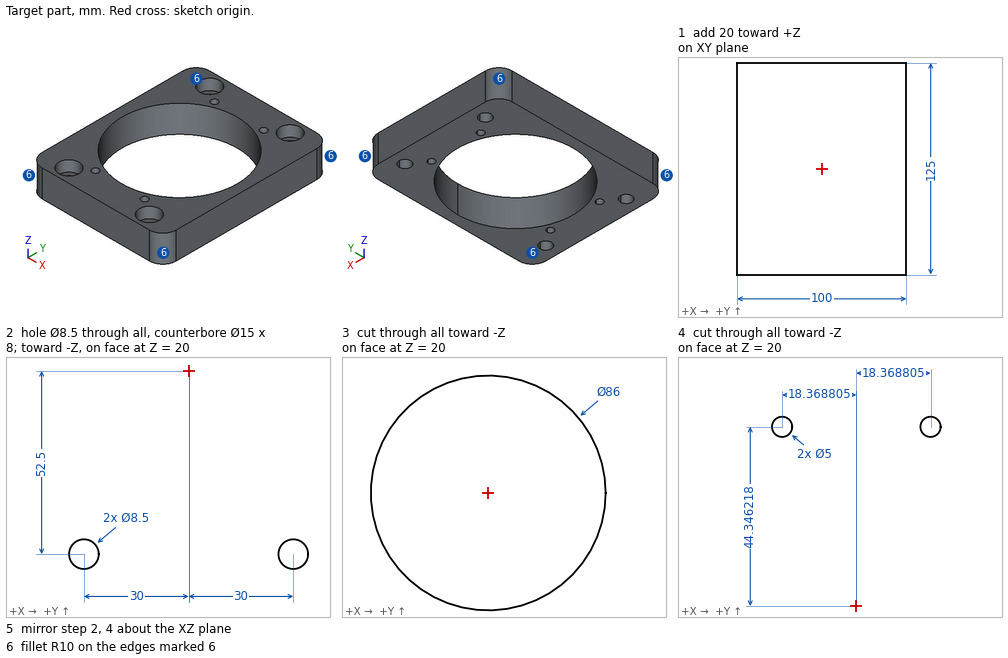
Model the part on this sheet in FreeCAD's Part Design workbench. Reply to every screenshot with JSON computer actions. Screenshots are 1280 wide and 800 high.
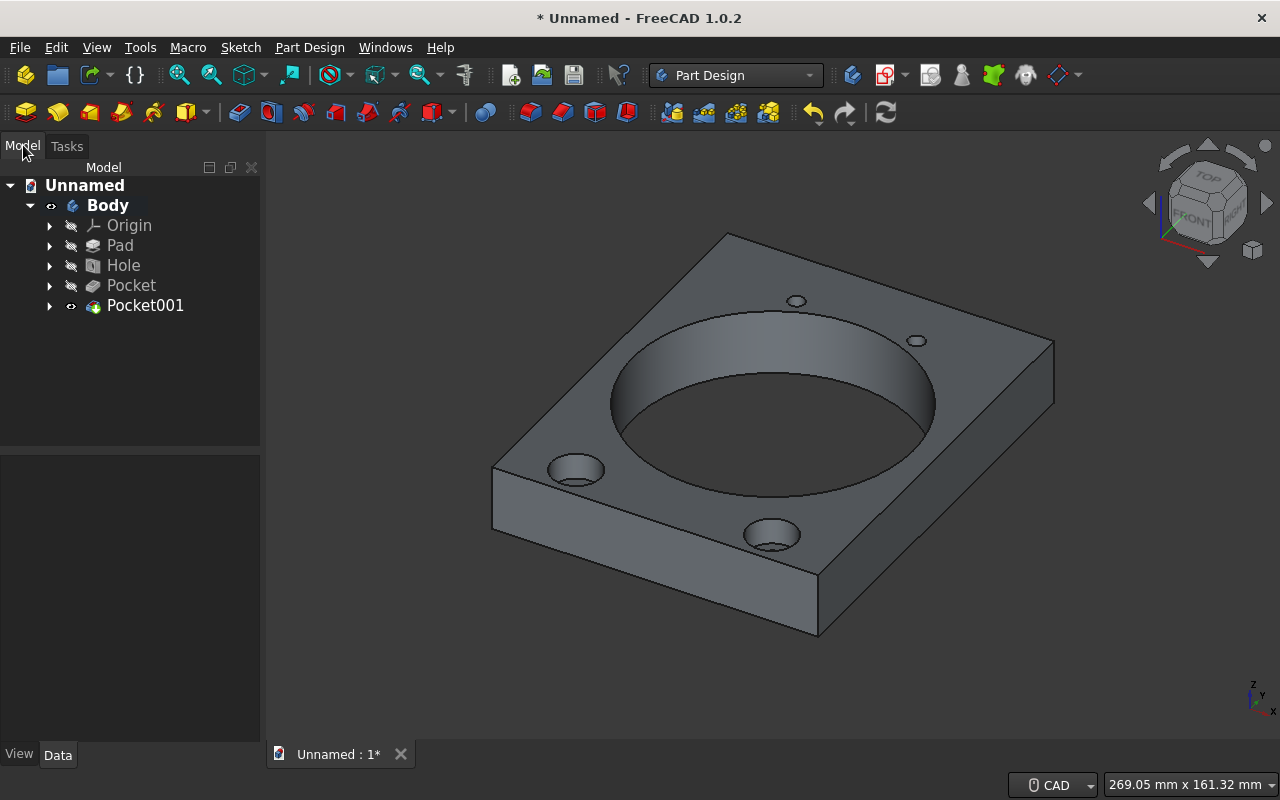
{"action": "left_click", "coordinate": [116, 266]}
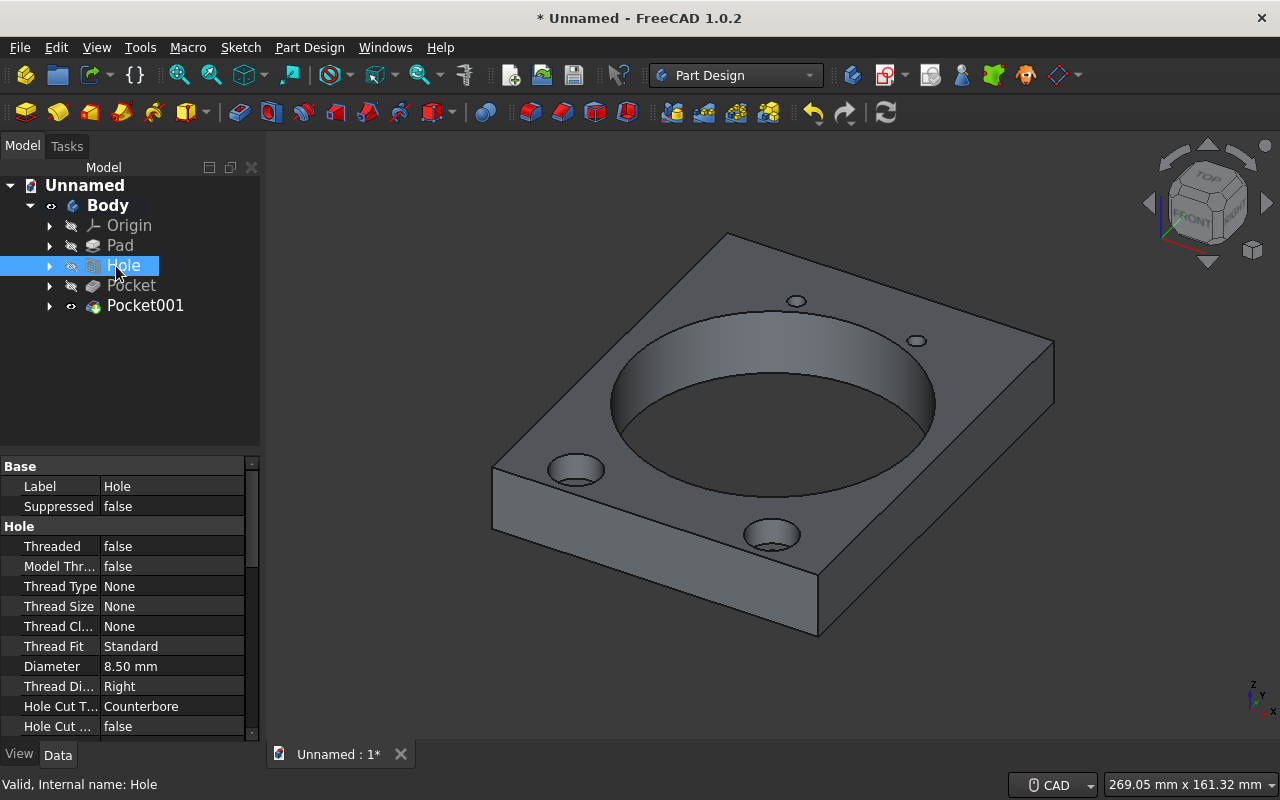
{"action": "left_click", "coordinate": [116, 306], "text": "ctrl"}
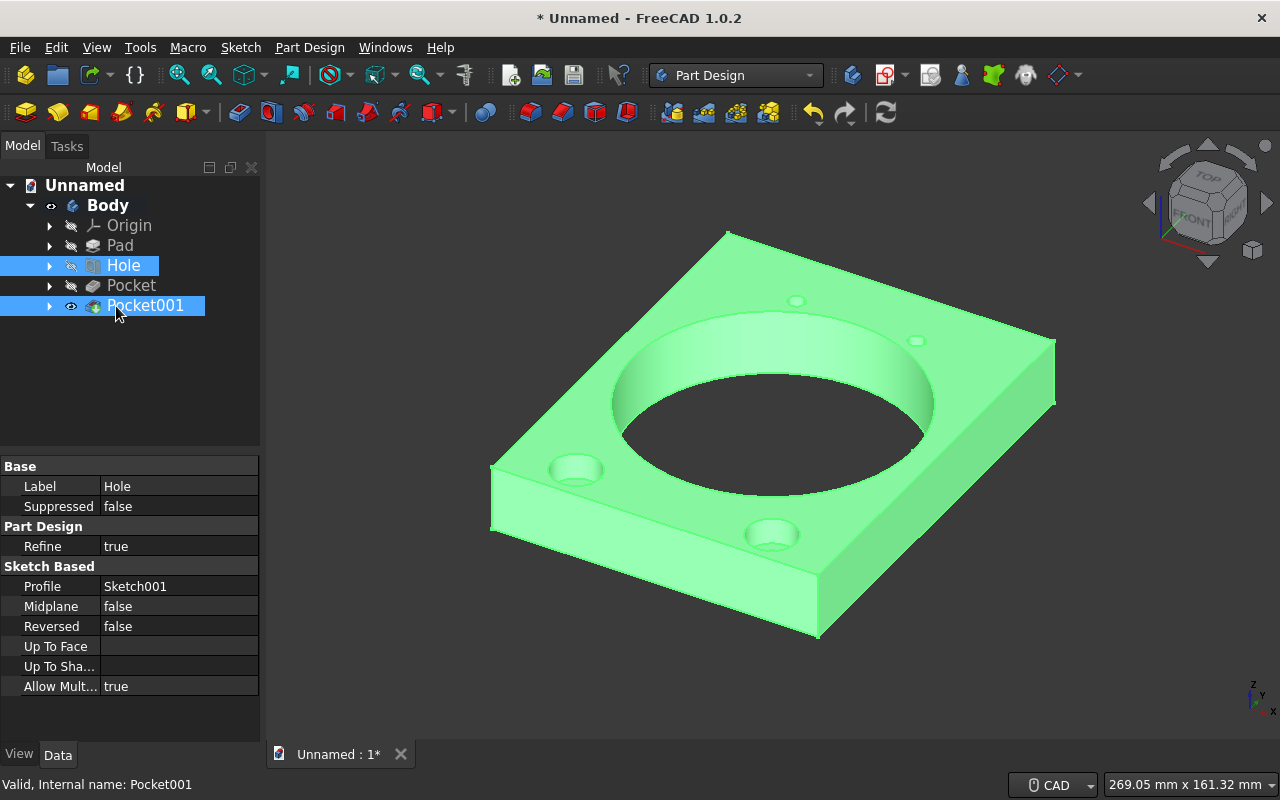
{"action": "left_click", "coordinate": [672, 112]}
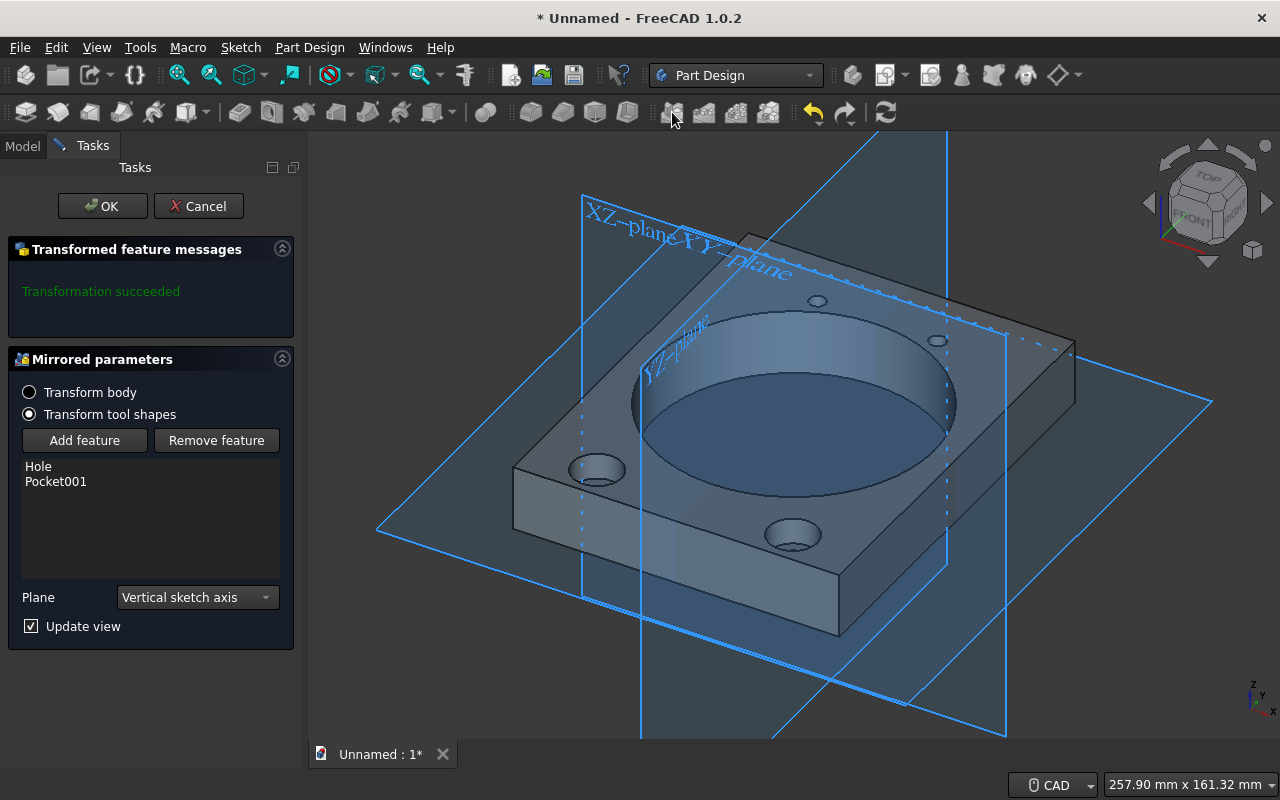
{"action": "left_click", "coordinate": [198, 598]}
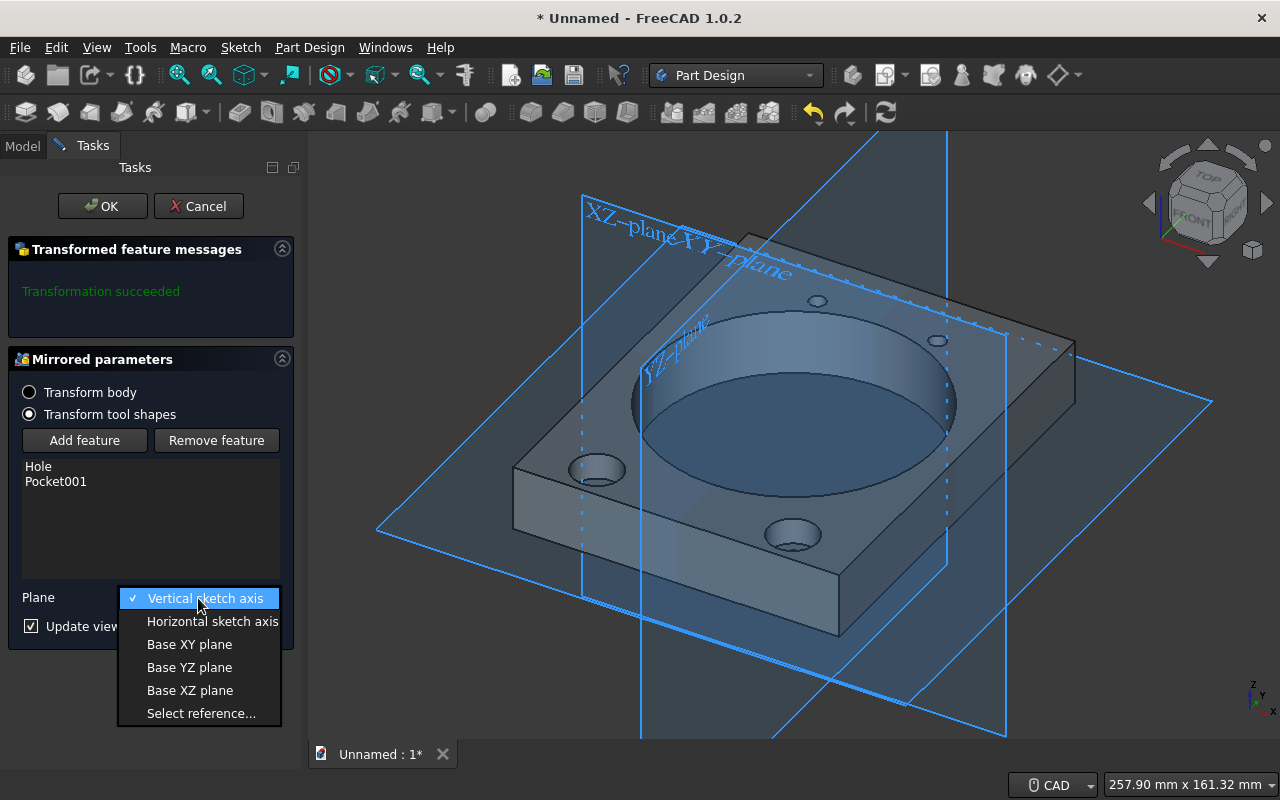
{"action": "left_click", "coordinate": [198, 690]}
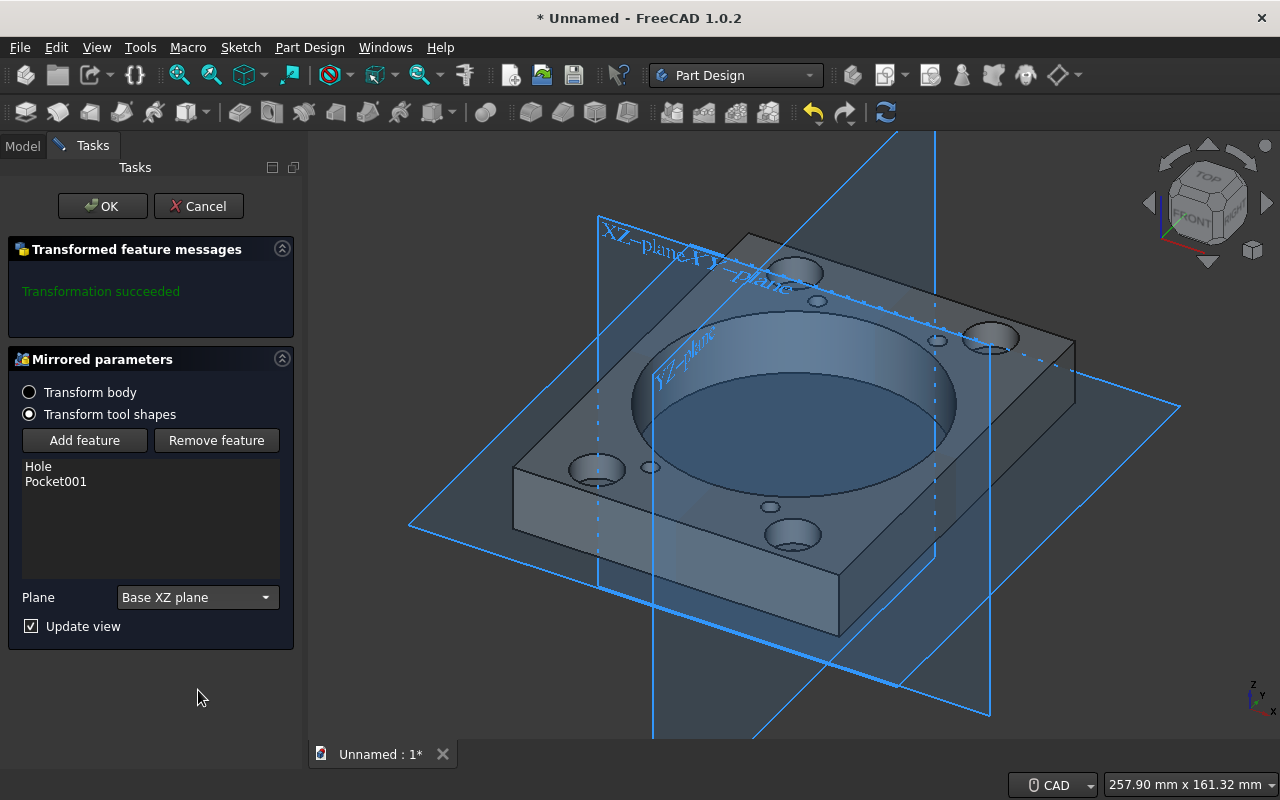
{"action": "left_click", "coordinate": [103, 206]}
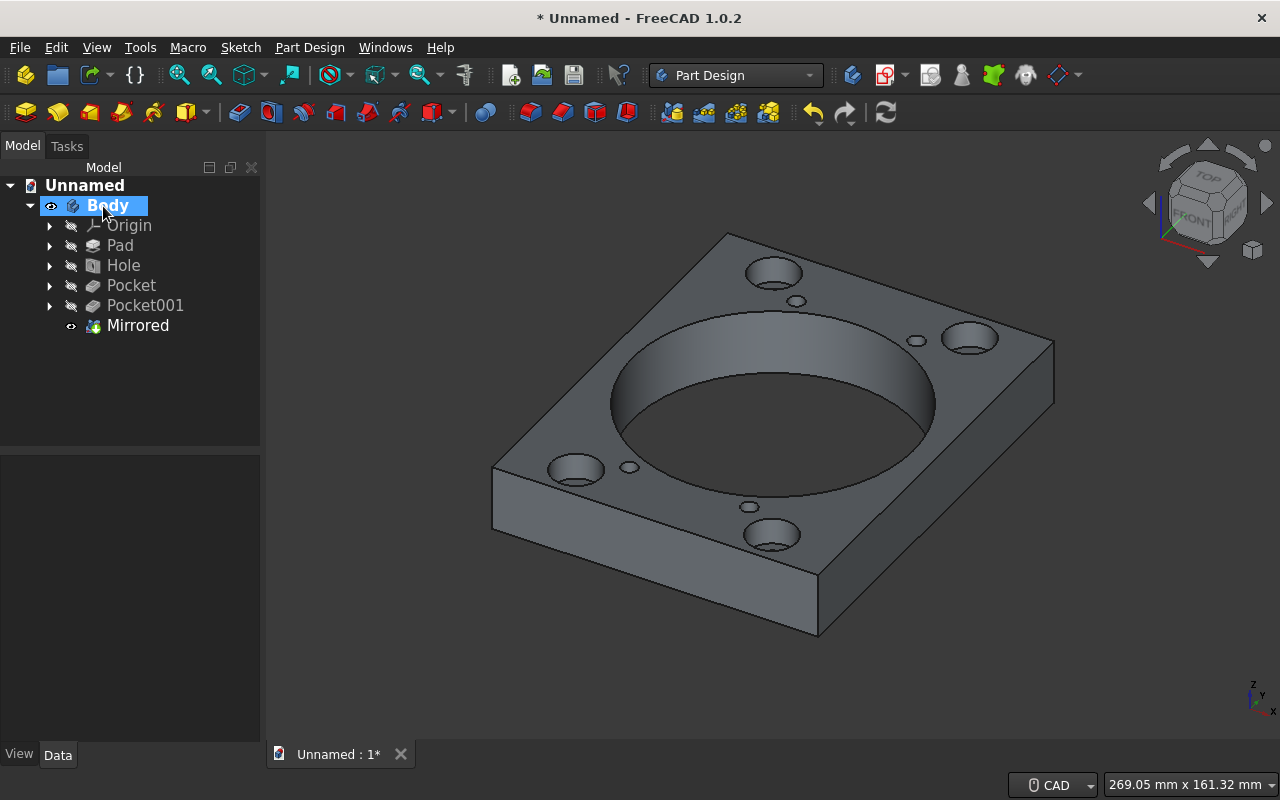
{"action": "left_click", "coordinate": [818, 605]}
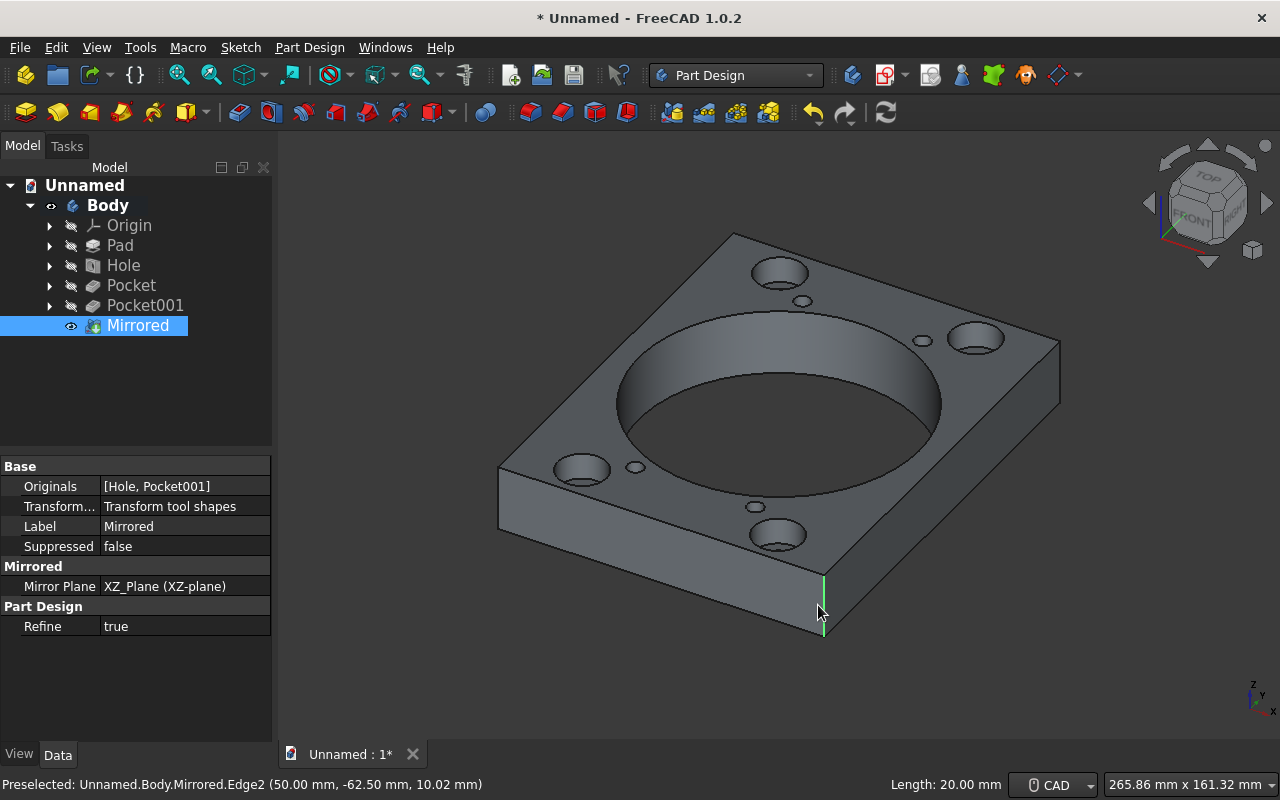
{"action": "key", "text": "0"}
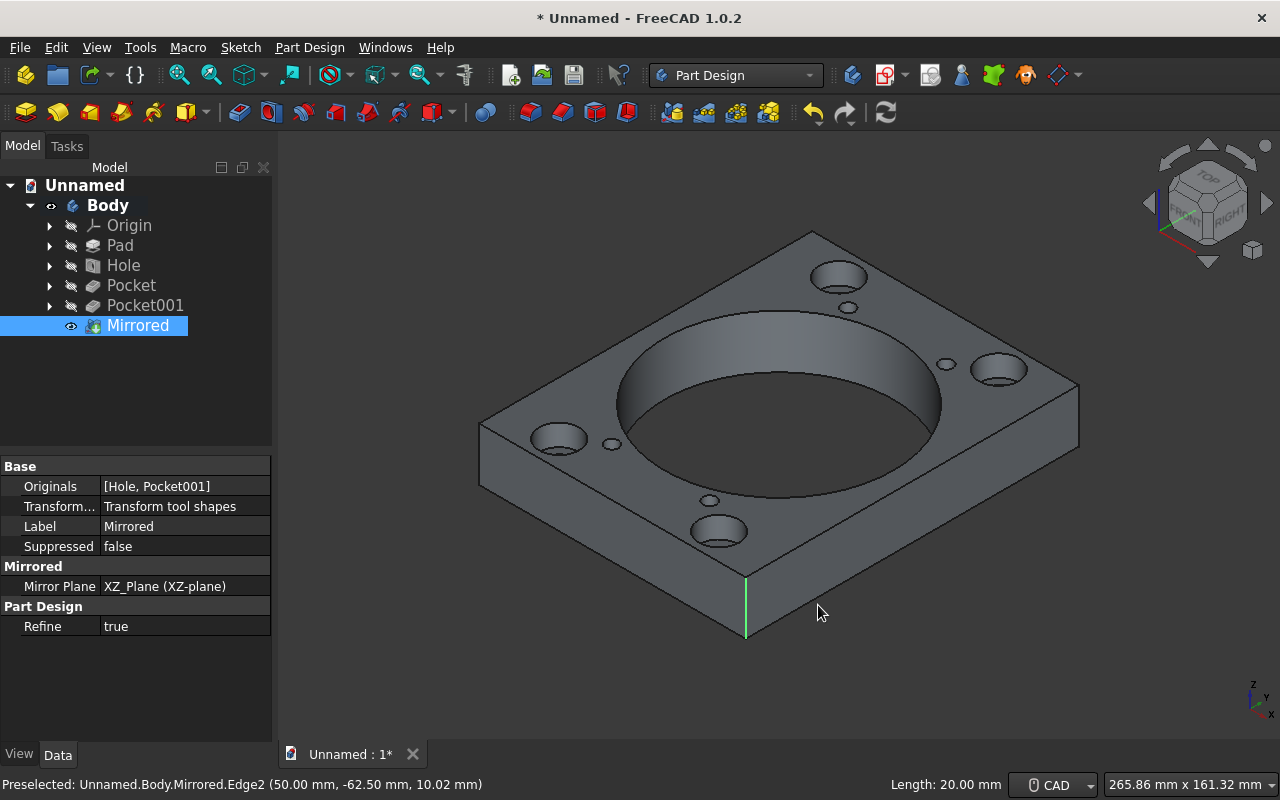
{"action": "key", "text": "2"}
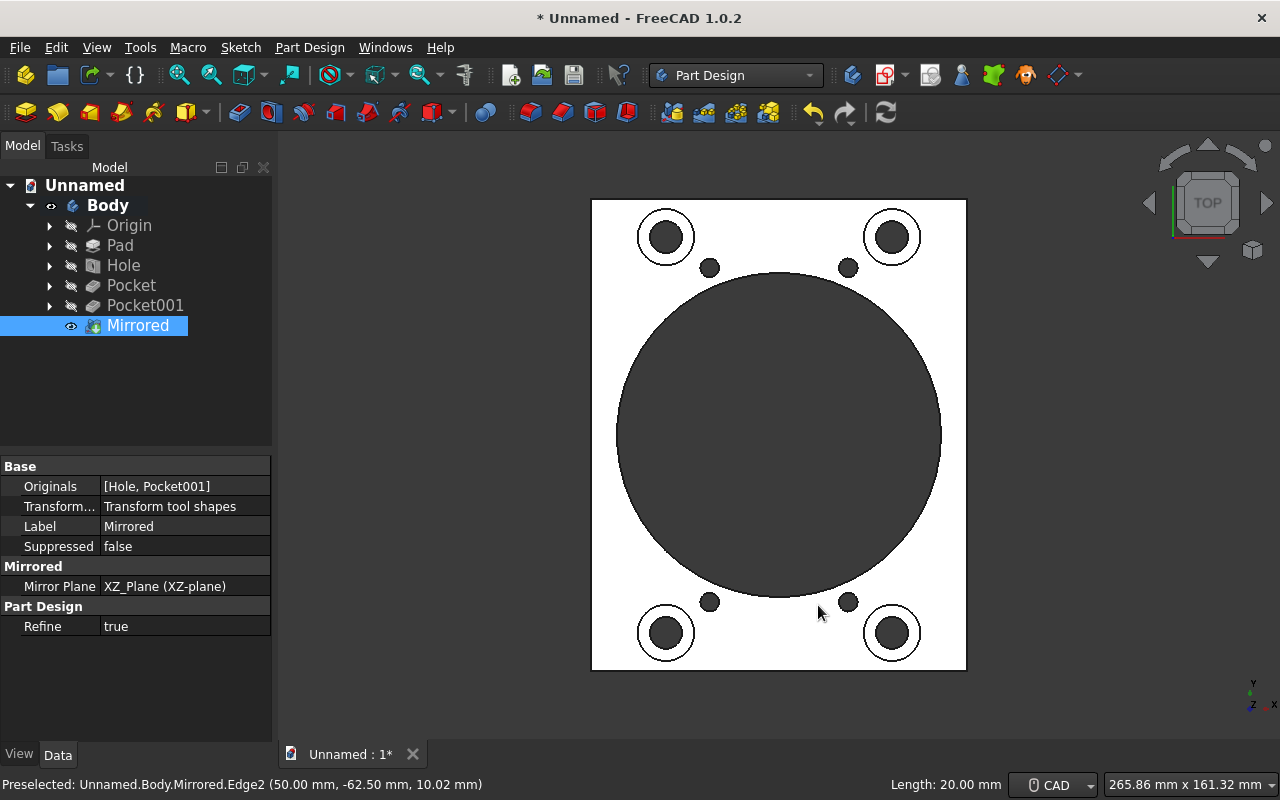
{"action": "key", "text": "1"}